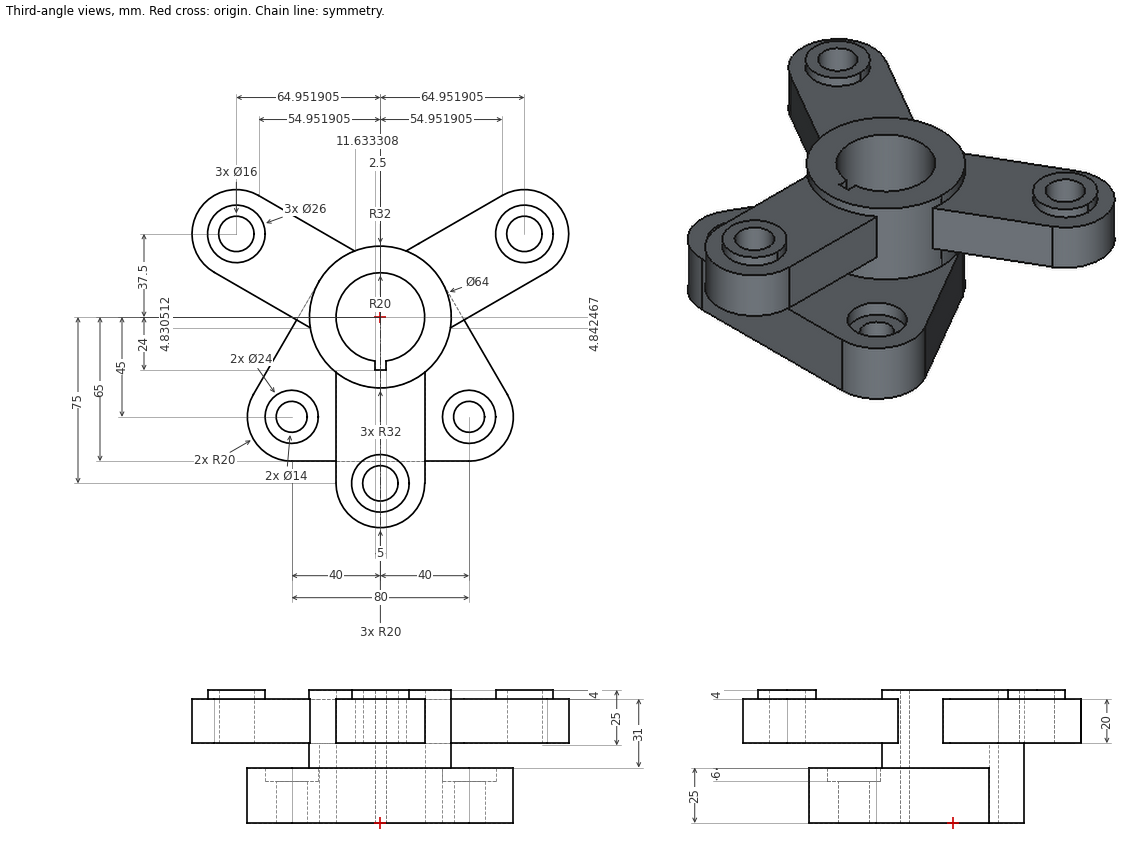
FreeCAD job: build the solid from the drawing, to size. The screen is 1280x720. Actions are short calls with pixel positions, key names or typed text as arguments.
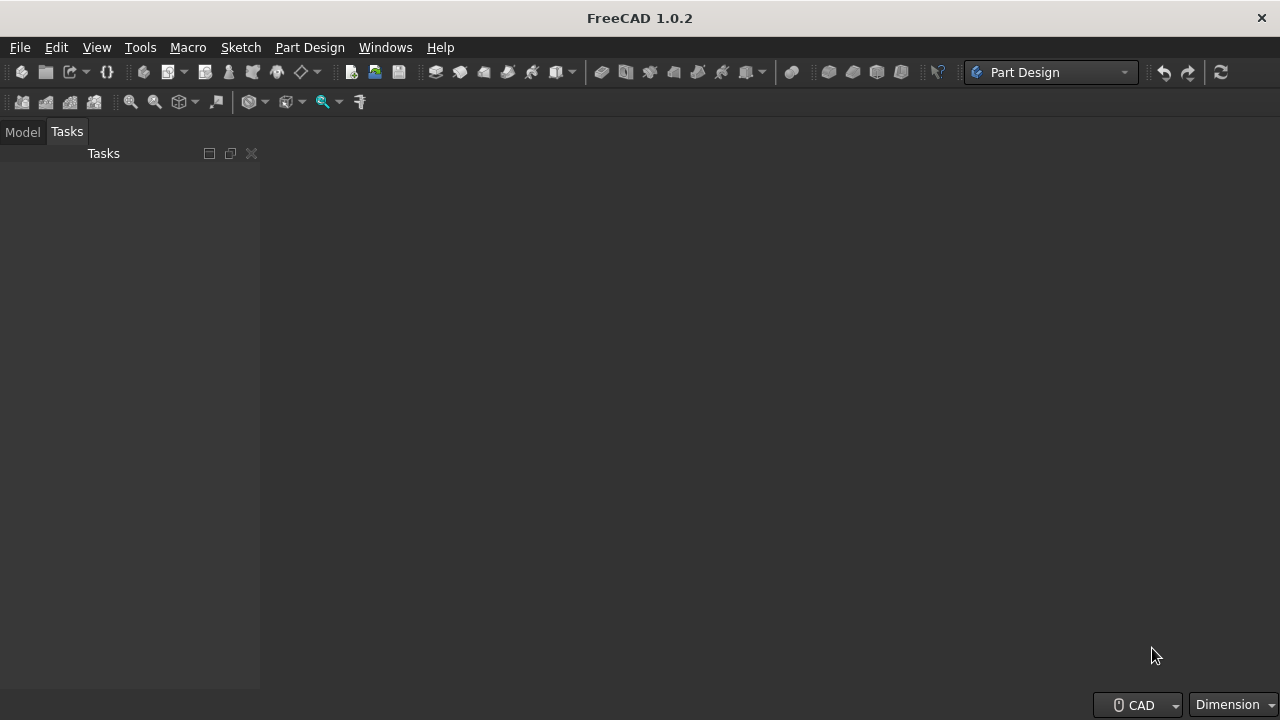
click(352, 72)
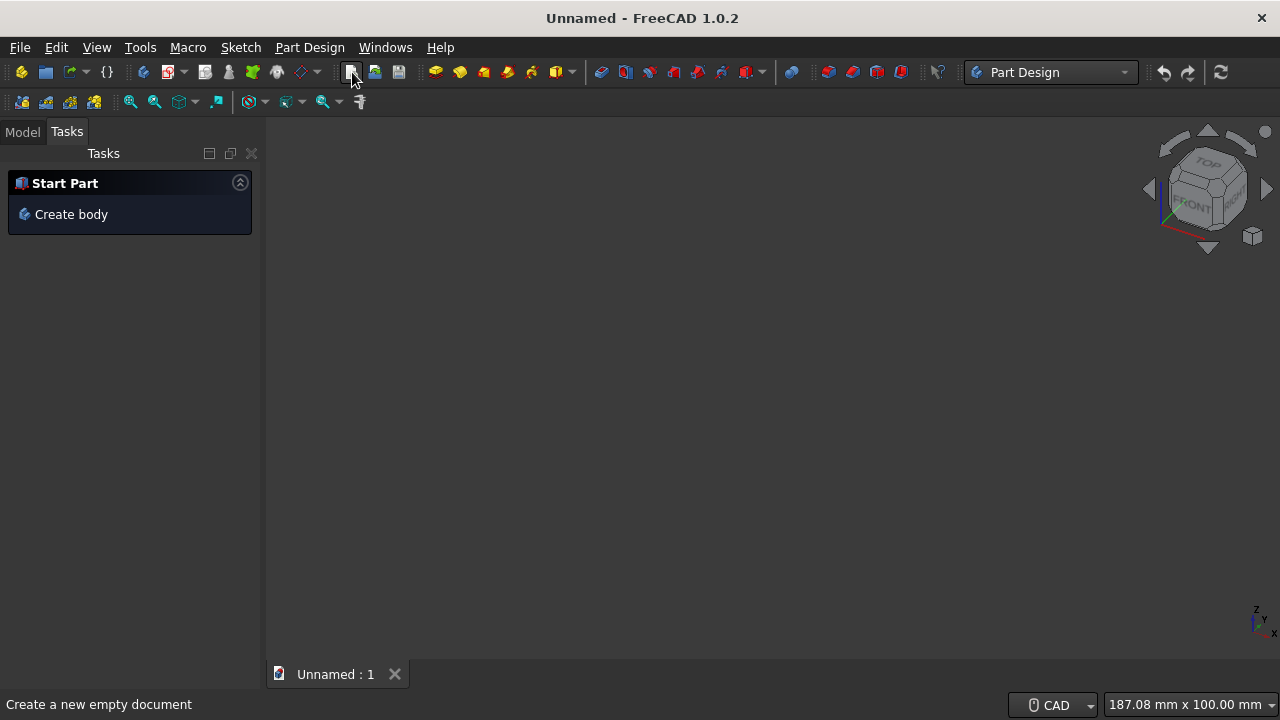
click(168, 72)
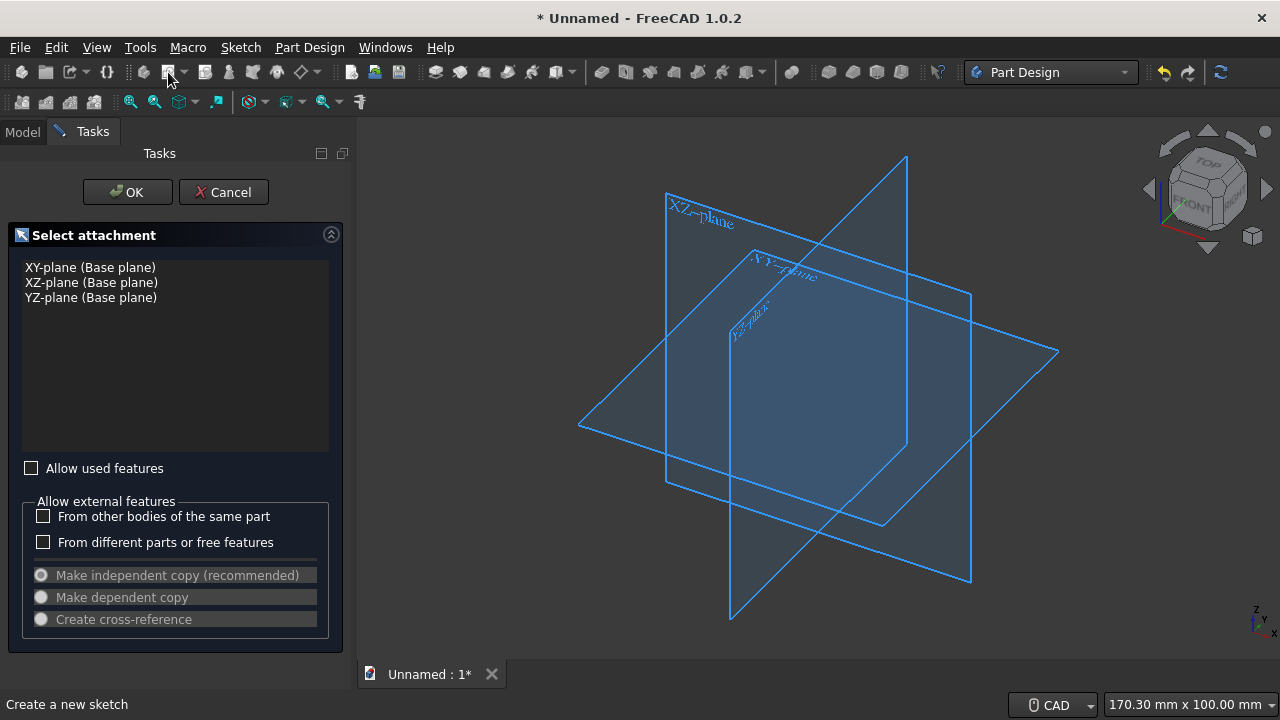
click(82, 268)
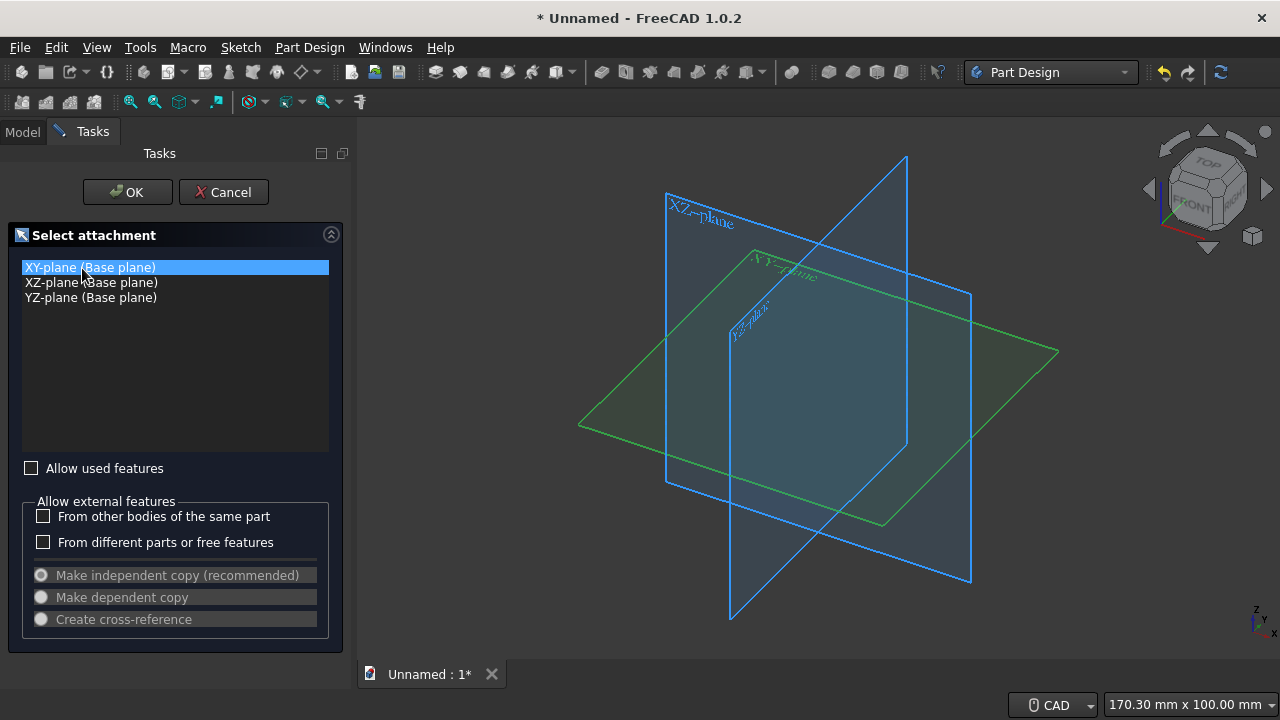
click(128, 192)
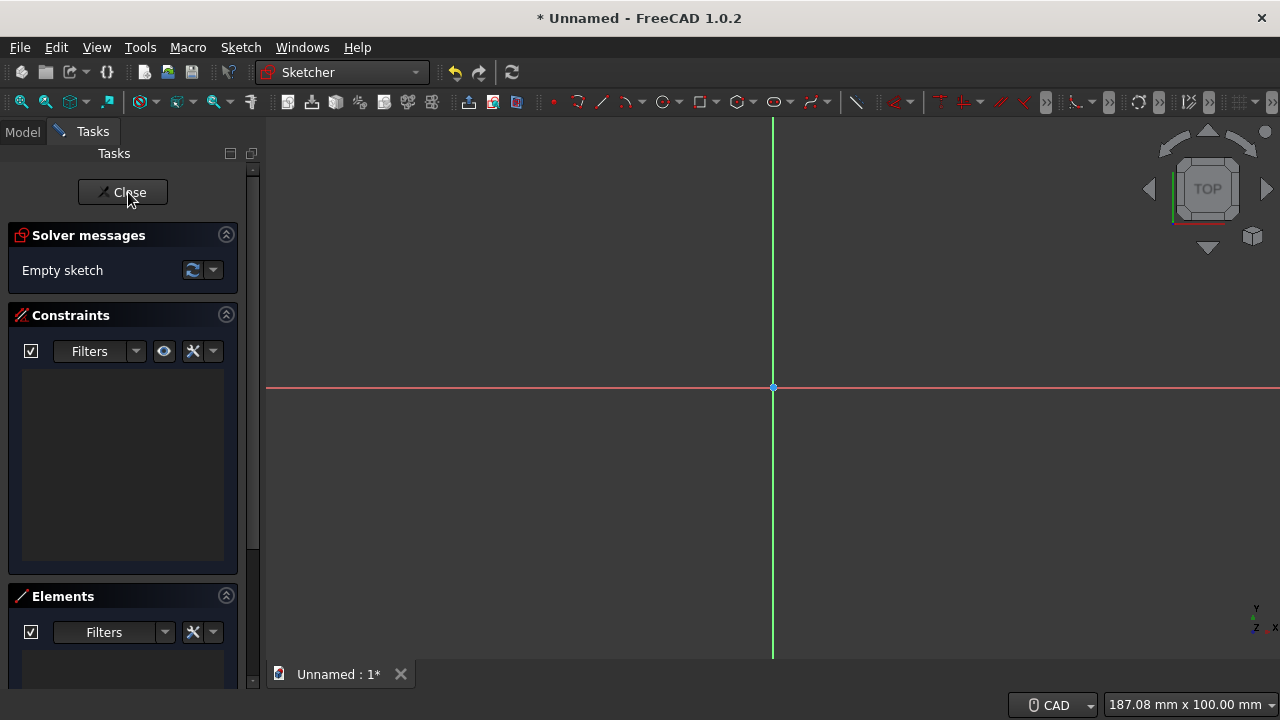
scroll(565, 206, down, 2)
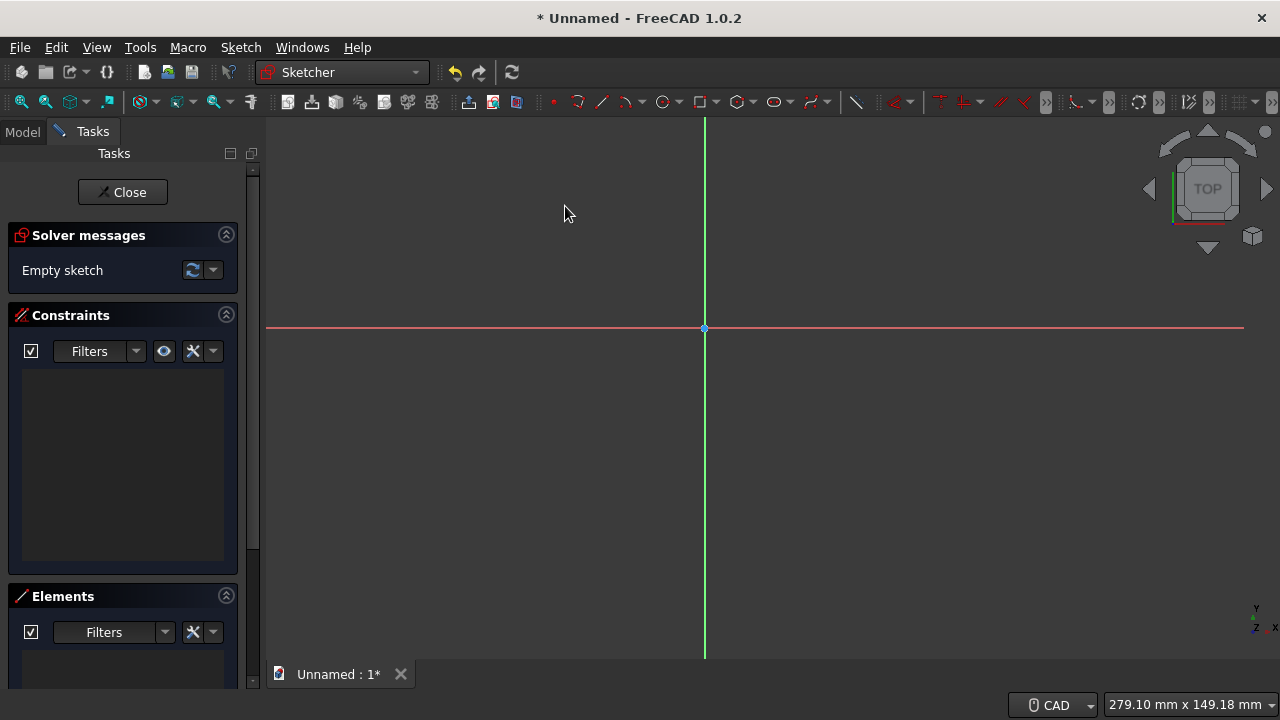
click(602, 102)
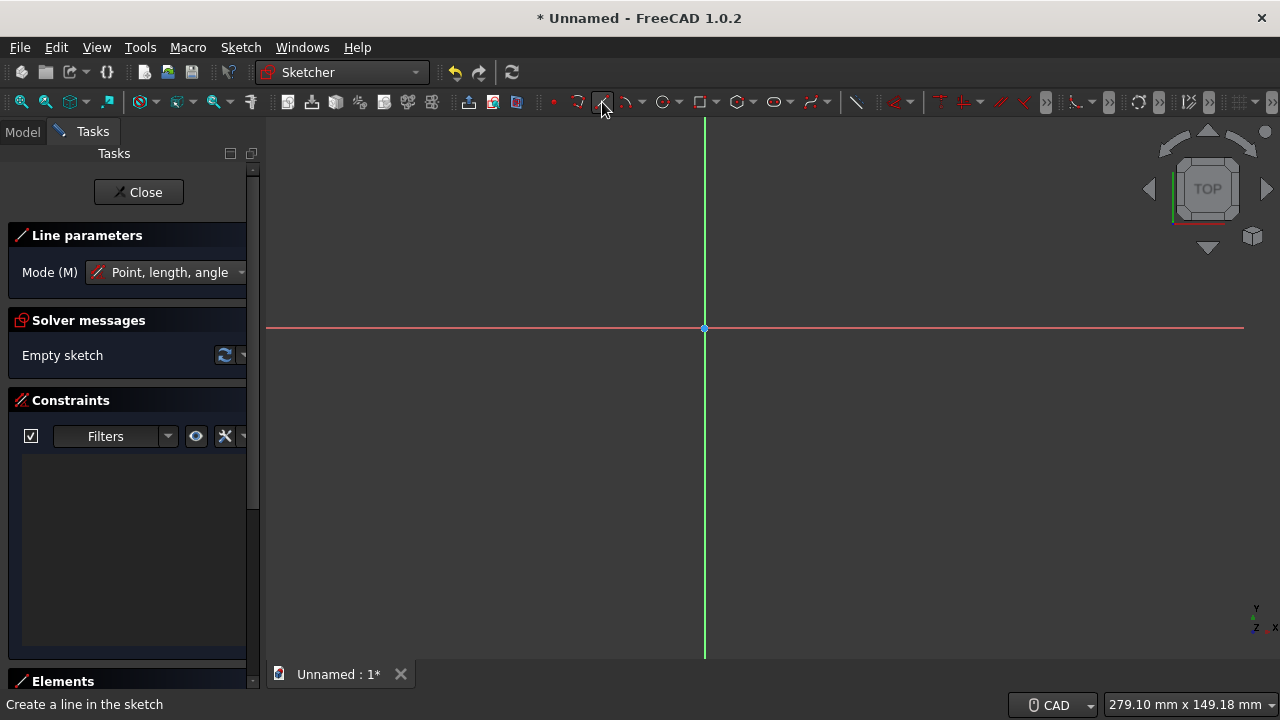
click(604, 270)
click(496, 455)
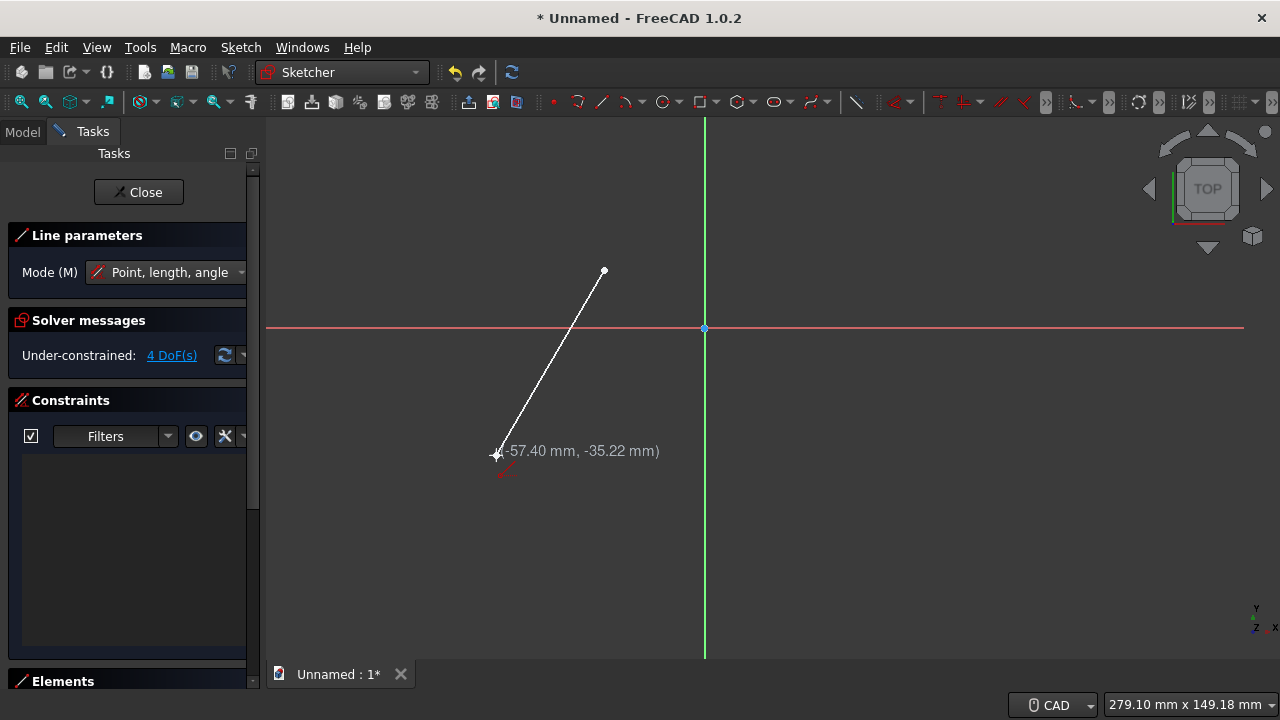
click(559, 564)
click(850, 564)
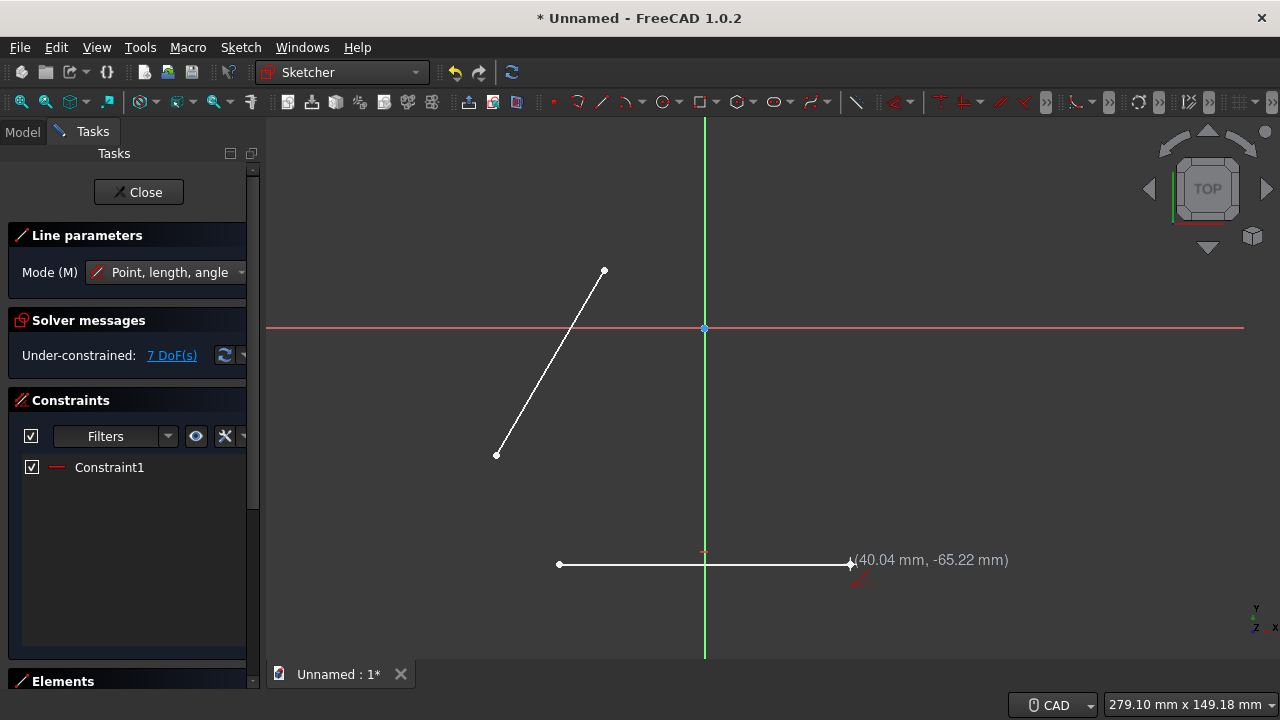
click(913, 455)
click(805, 270)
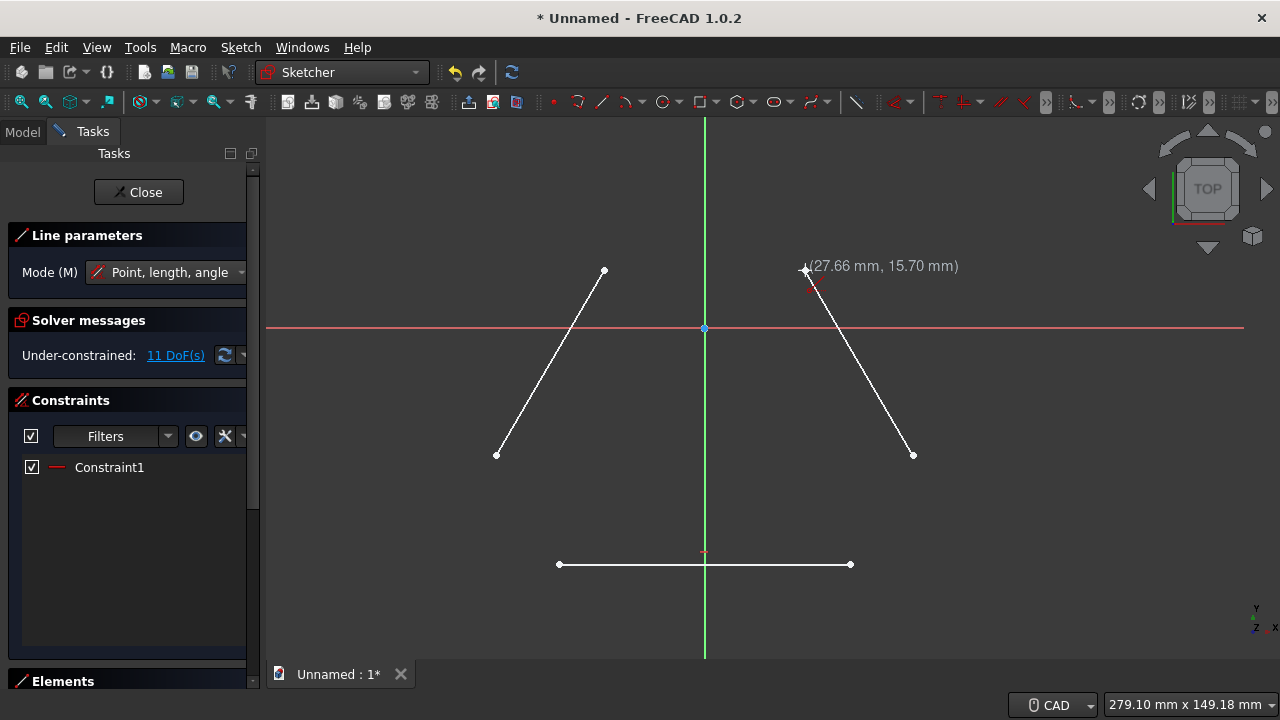
key(g)
key(3)
key(a)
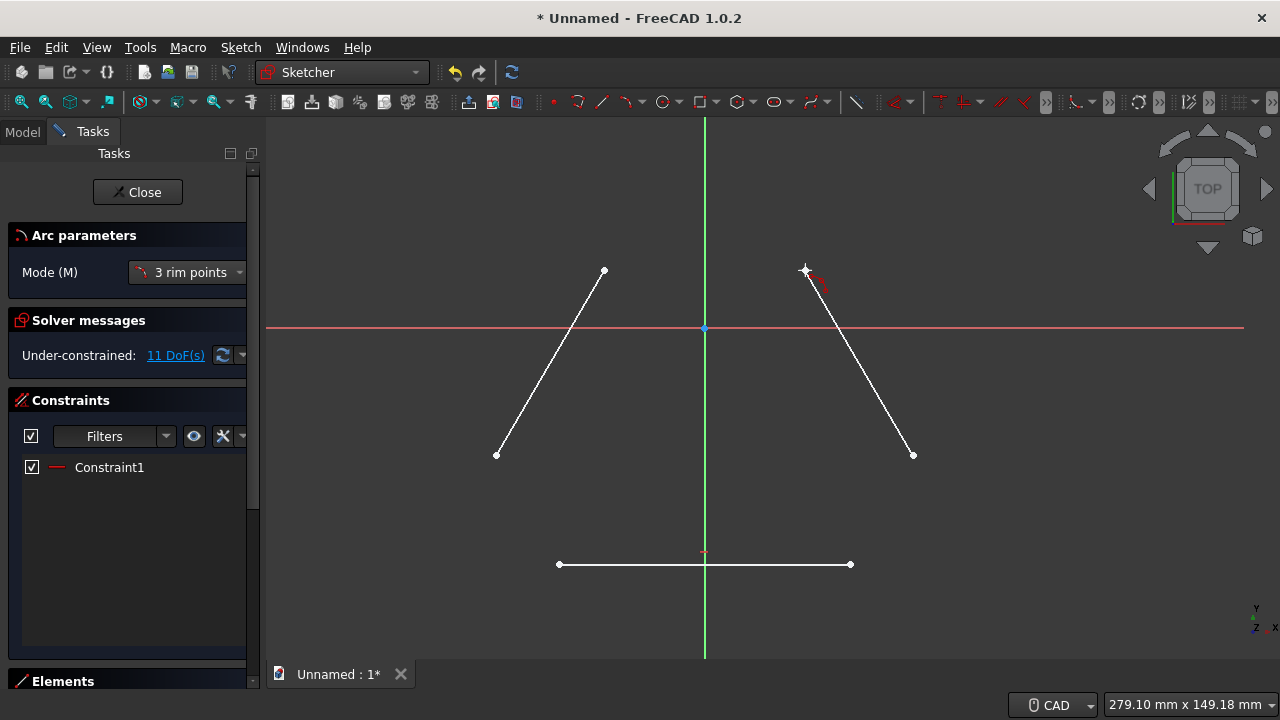
click(496, 456)
click(559, 565)
click(496, 528)